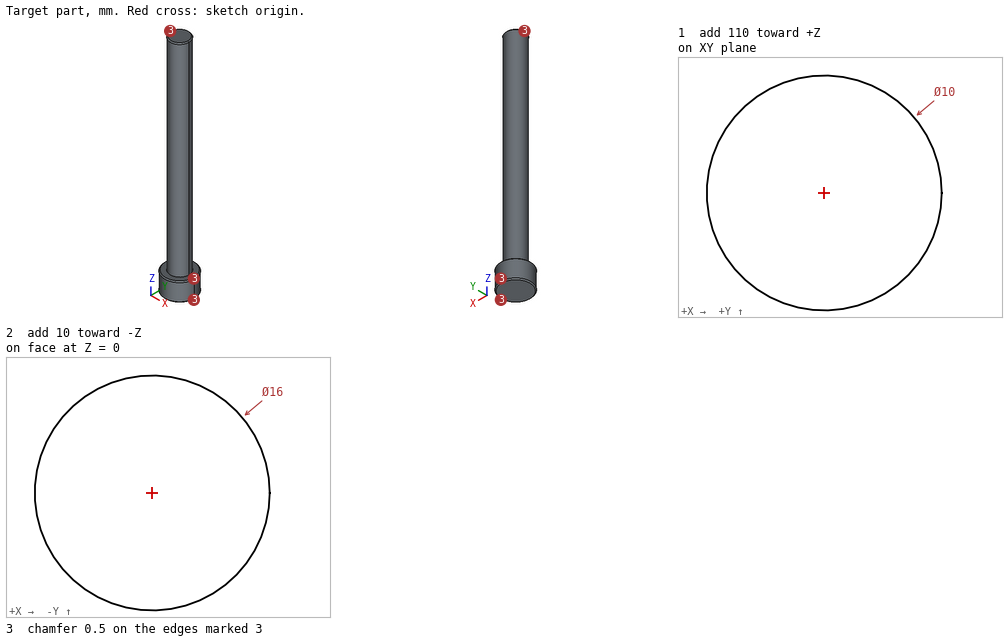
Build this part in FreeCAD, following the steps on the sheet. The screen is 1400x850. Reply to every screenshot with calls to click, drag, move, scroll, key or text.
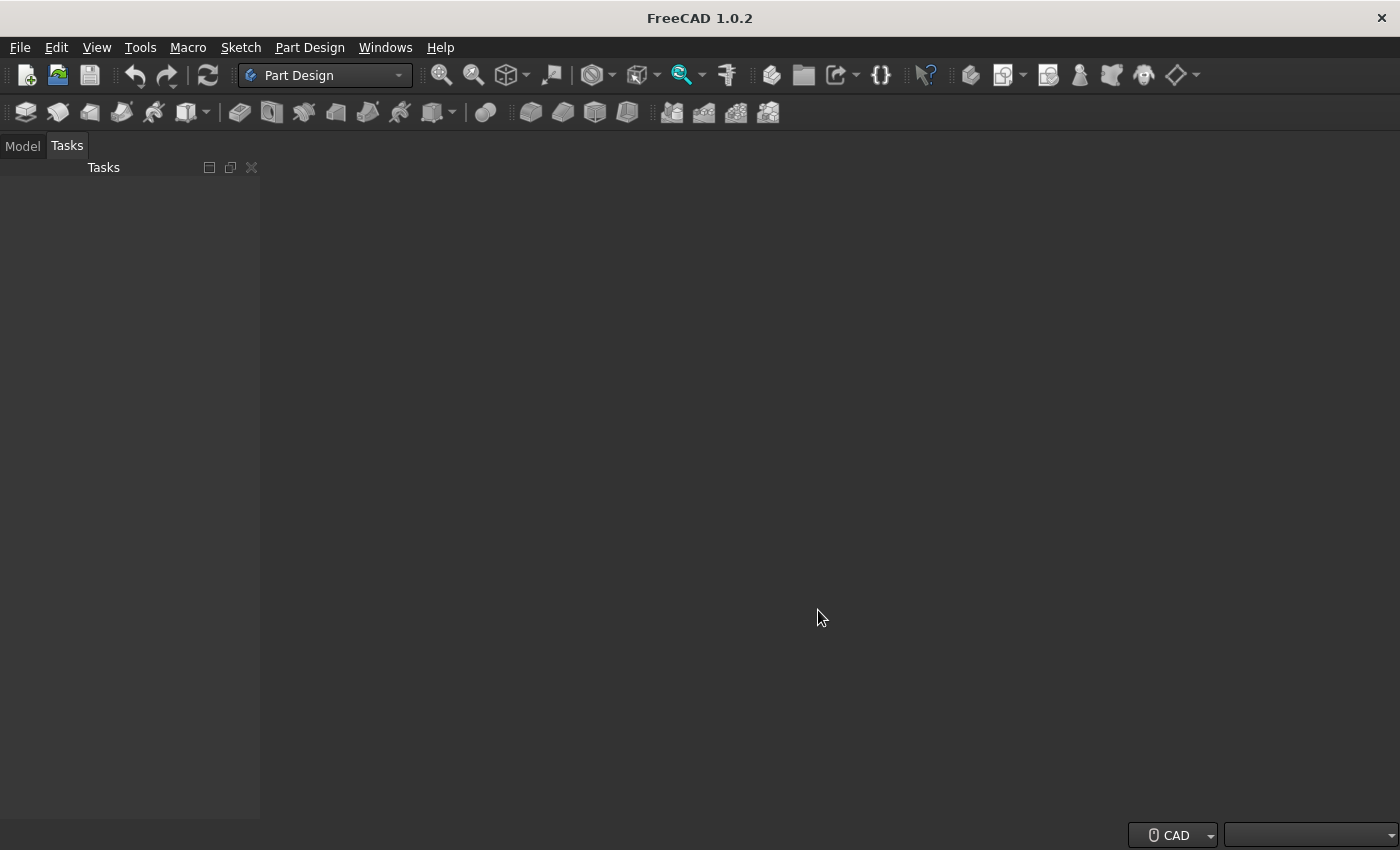
key(ctrl+n)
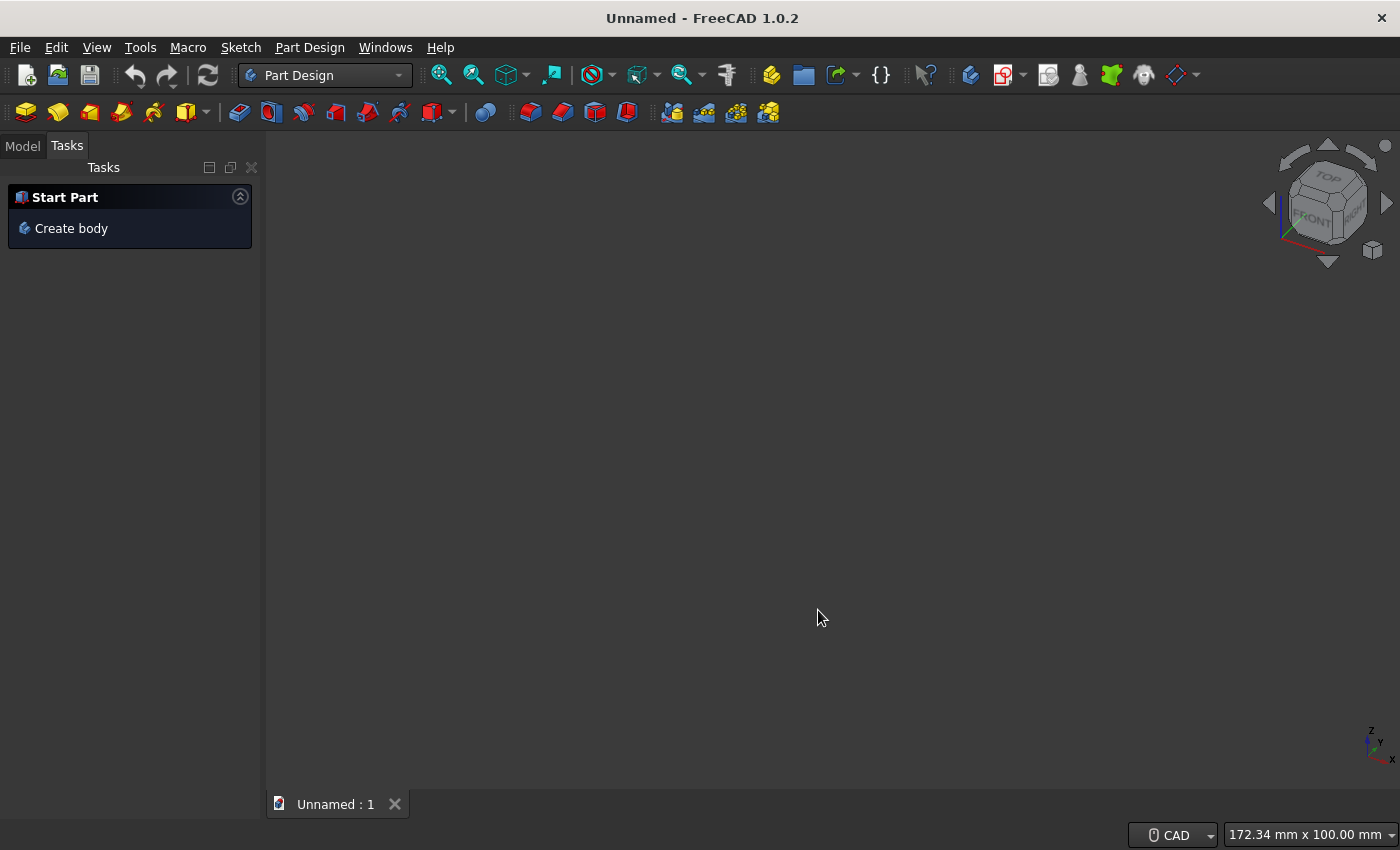
click(1004, 76)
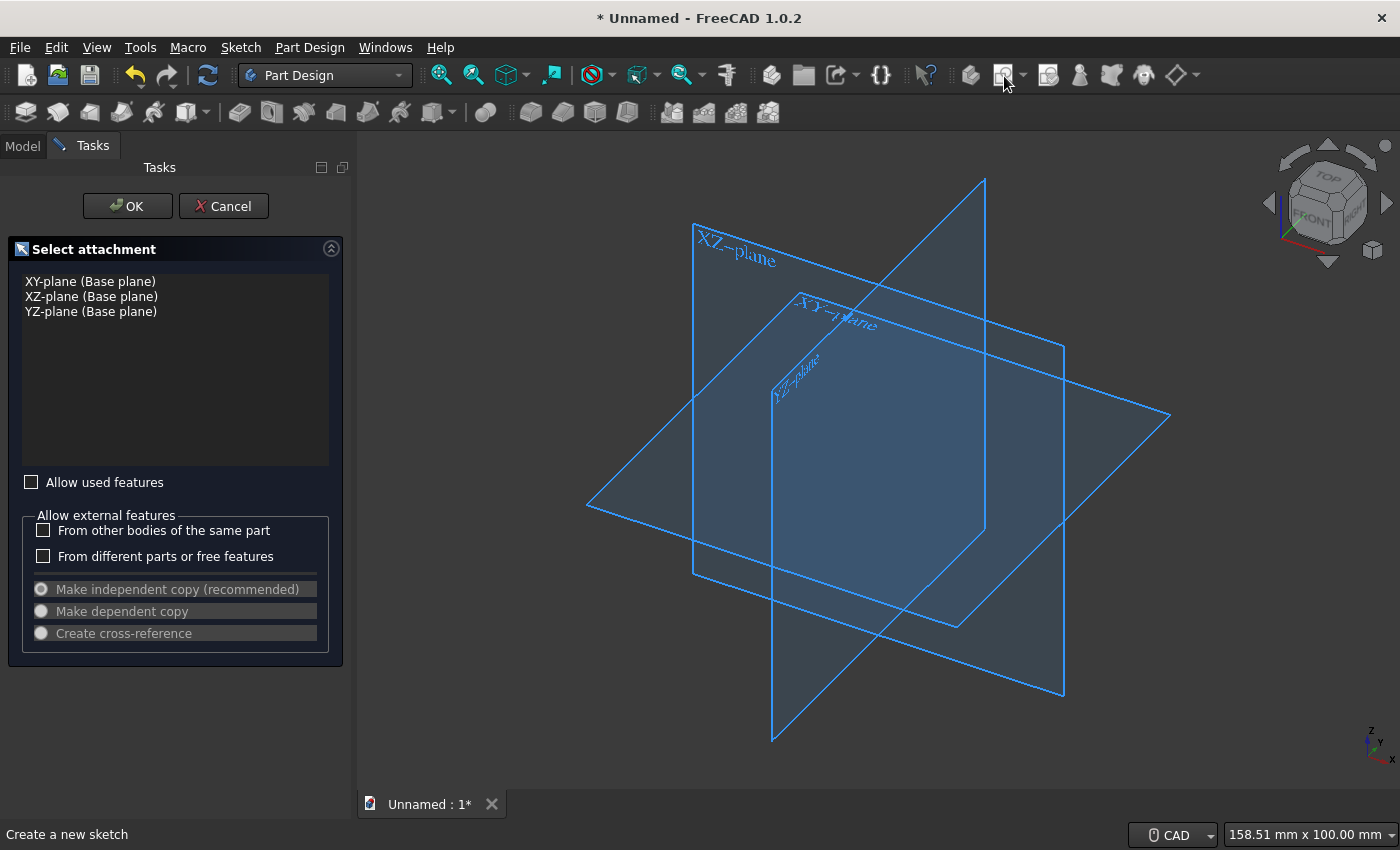
click(82, 282)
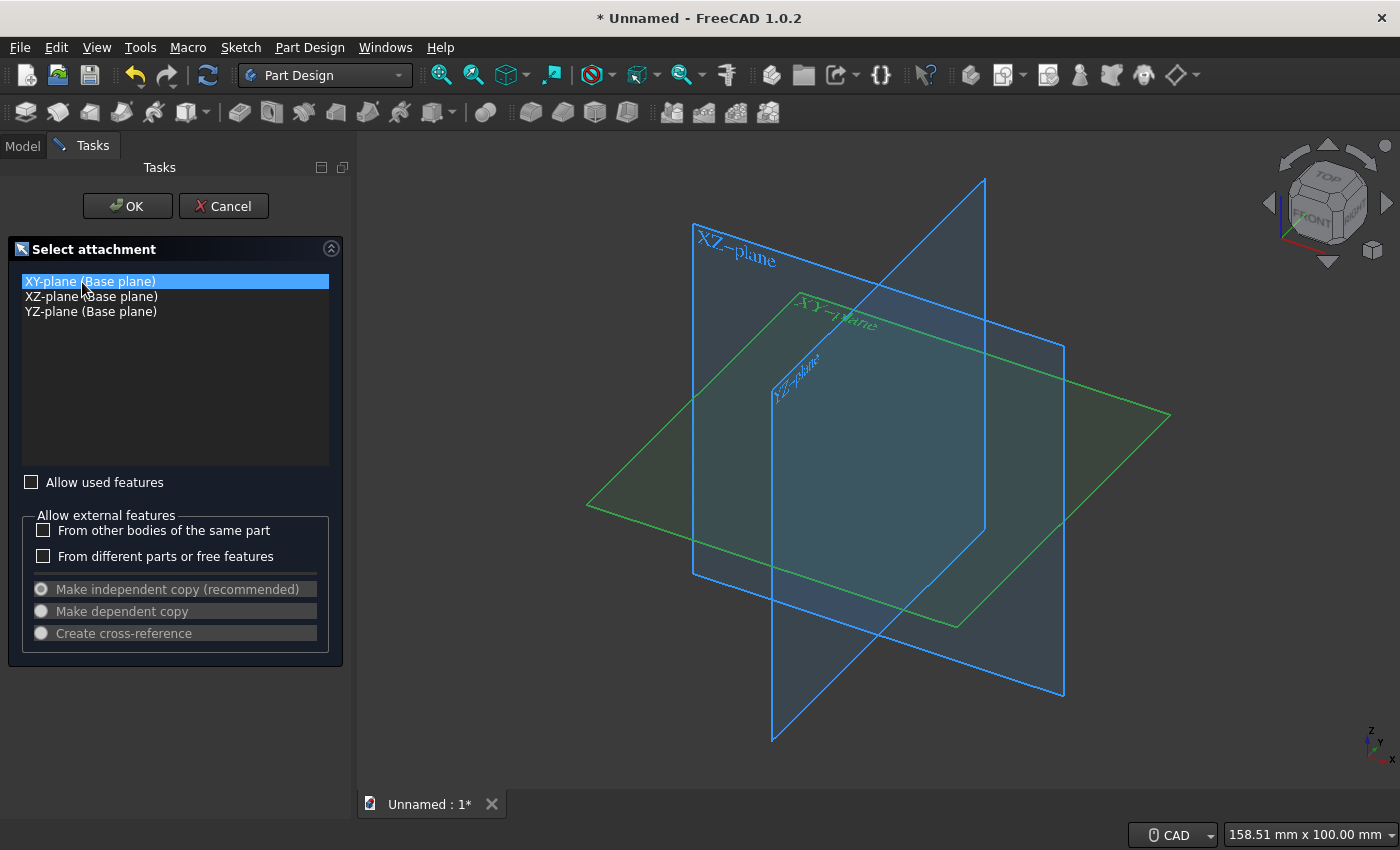
click(128, 206)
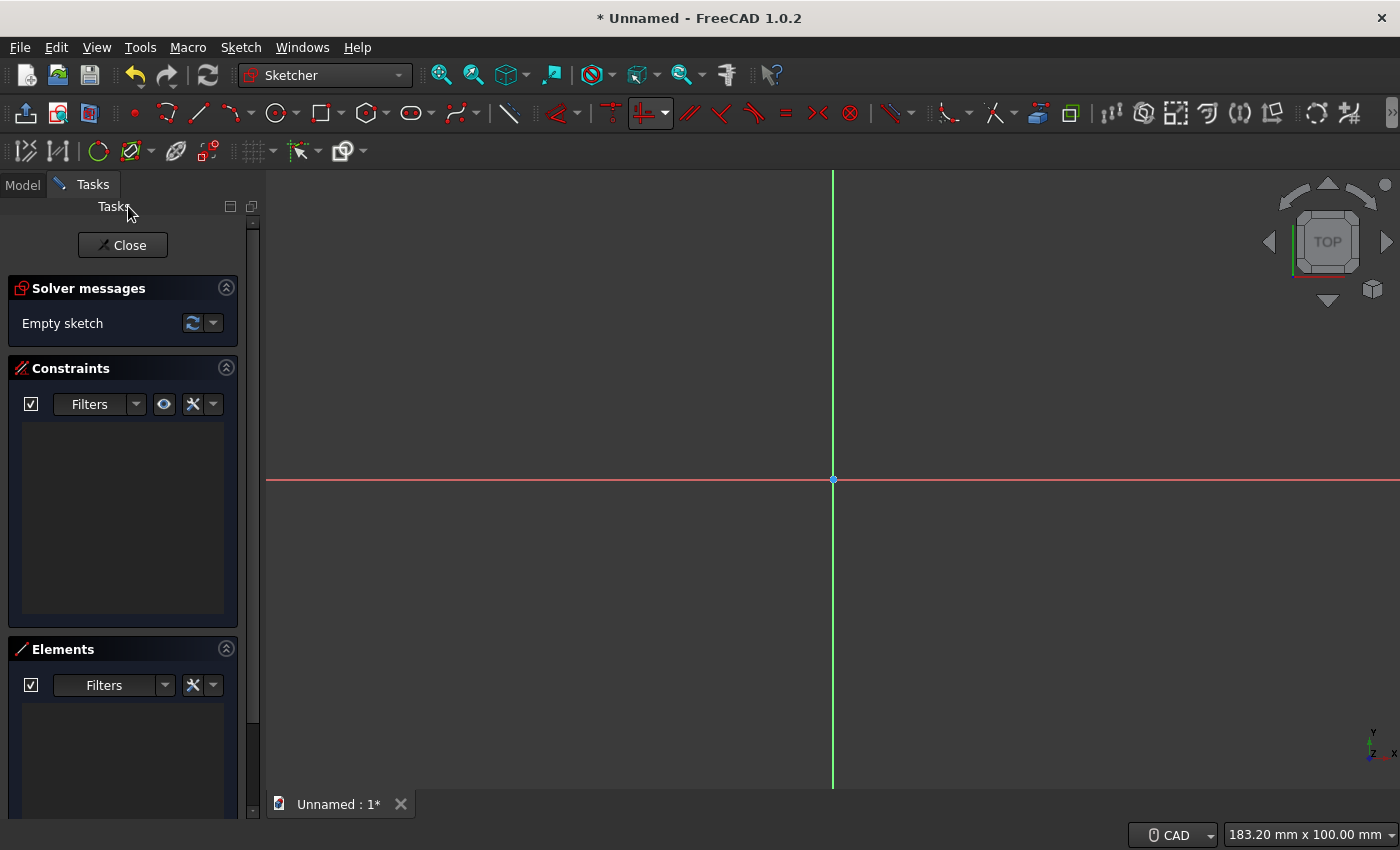
scroll(847, 480, up, 9)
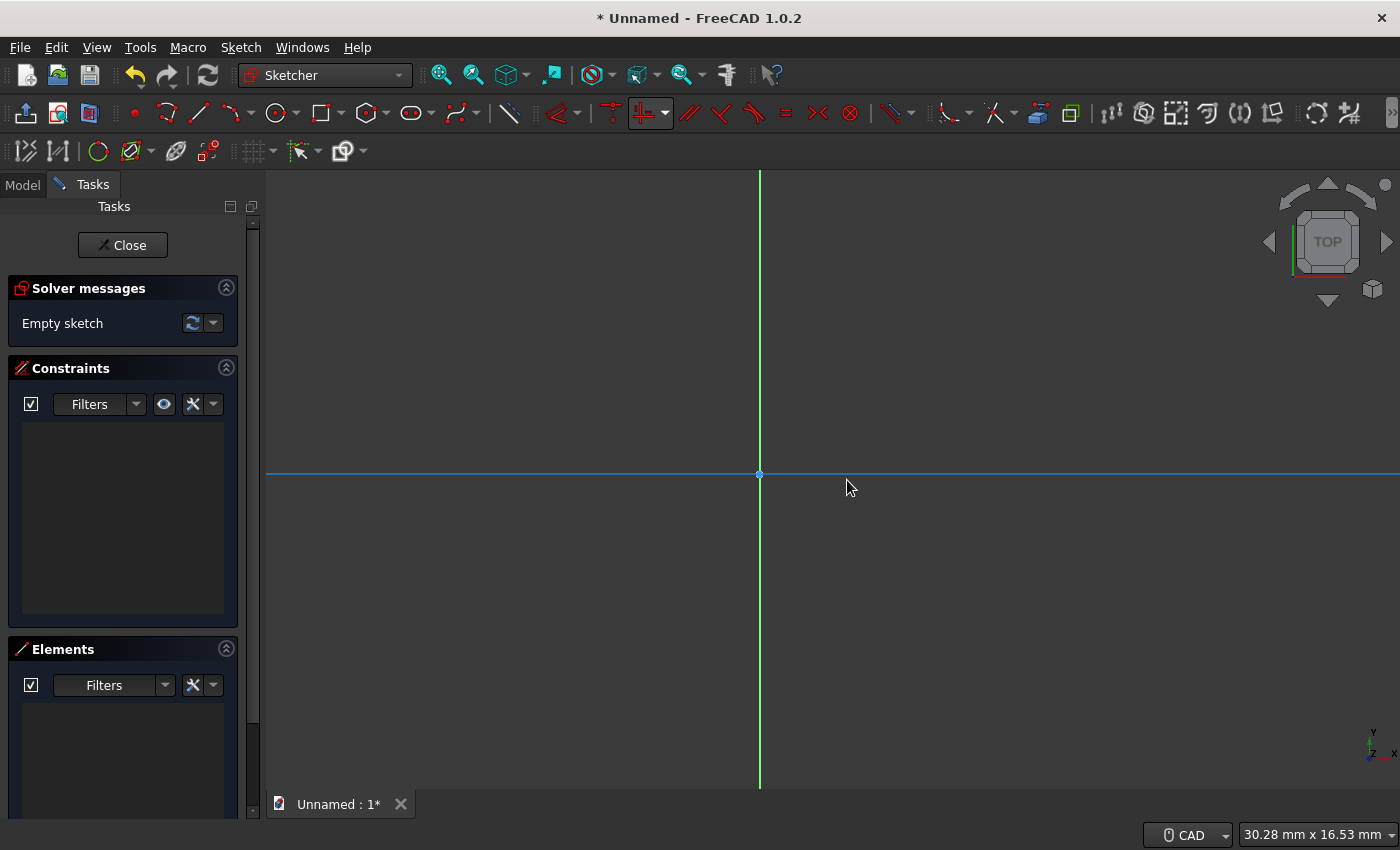
click(276, 114)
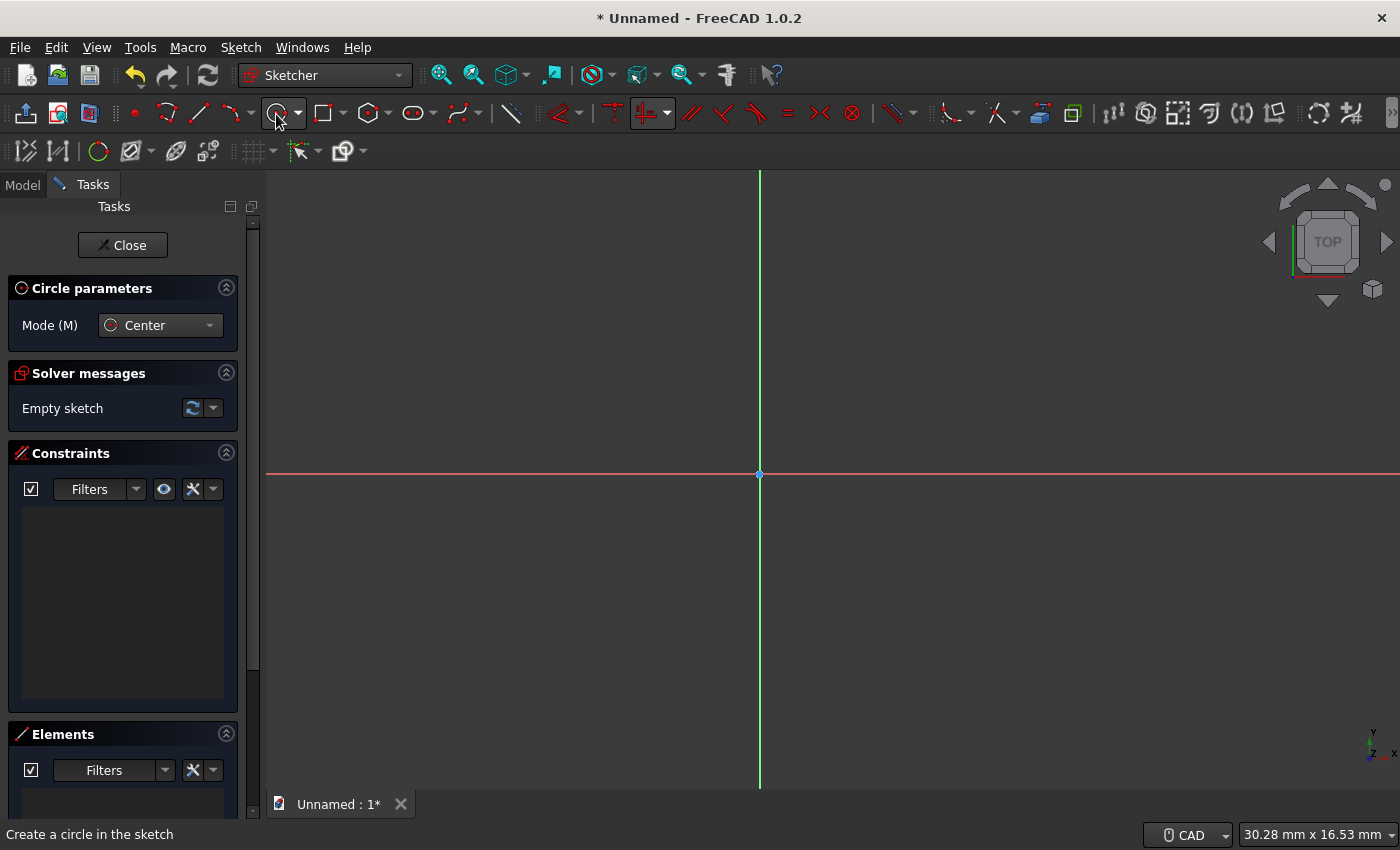
click(760, 474)
click(892, 342)
key(Escape)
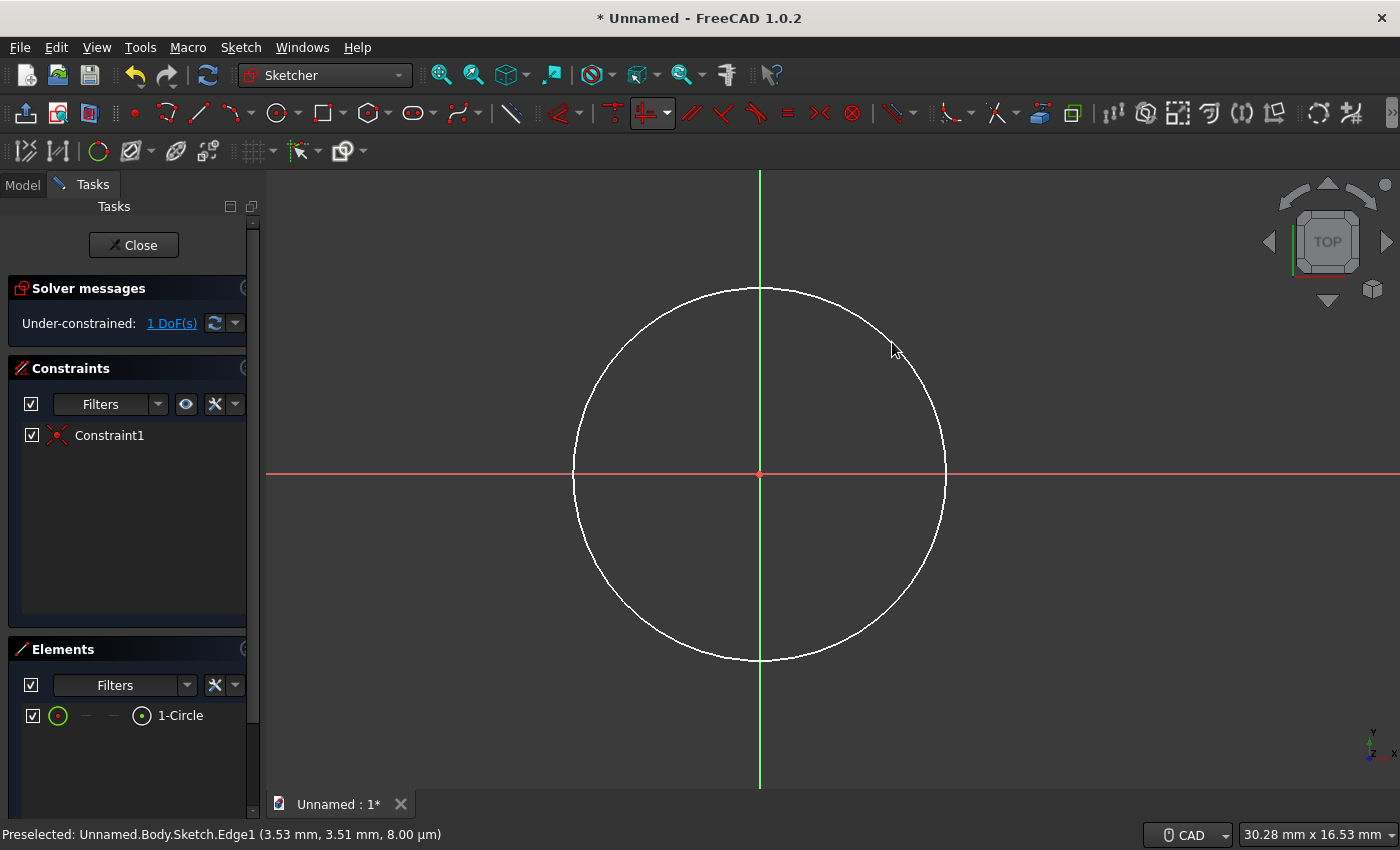
click(891, 342)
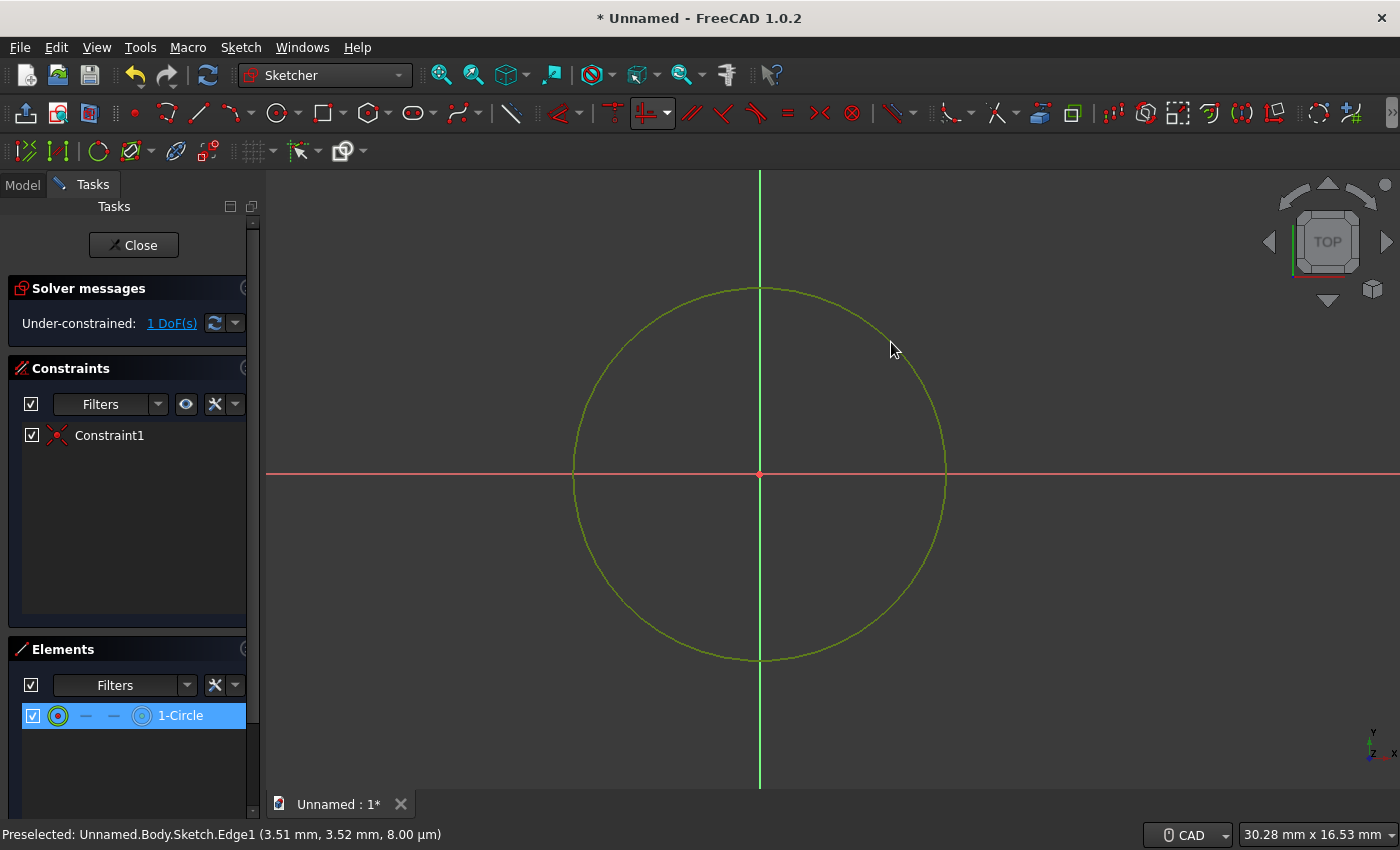
key(k)
key(o)